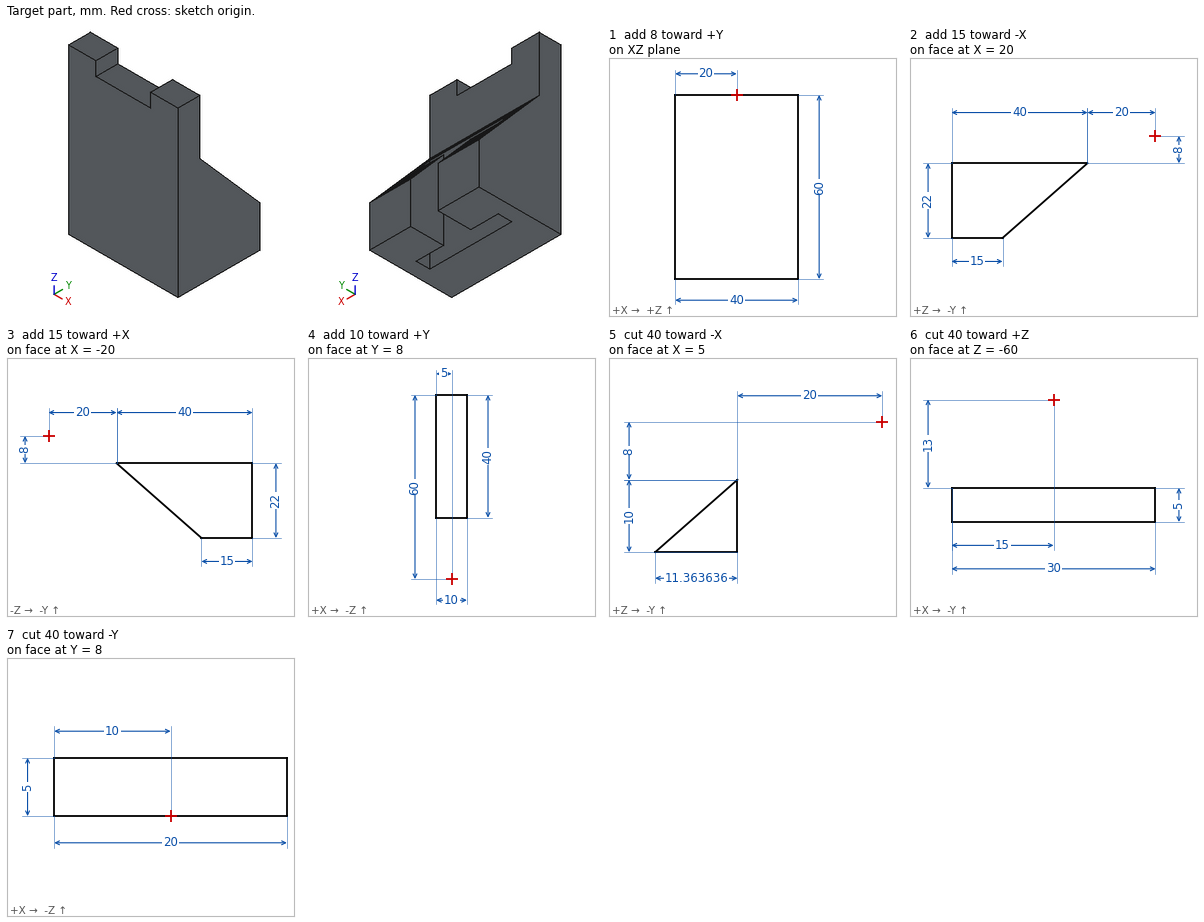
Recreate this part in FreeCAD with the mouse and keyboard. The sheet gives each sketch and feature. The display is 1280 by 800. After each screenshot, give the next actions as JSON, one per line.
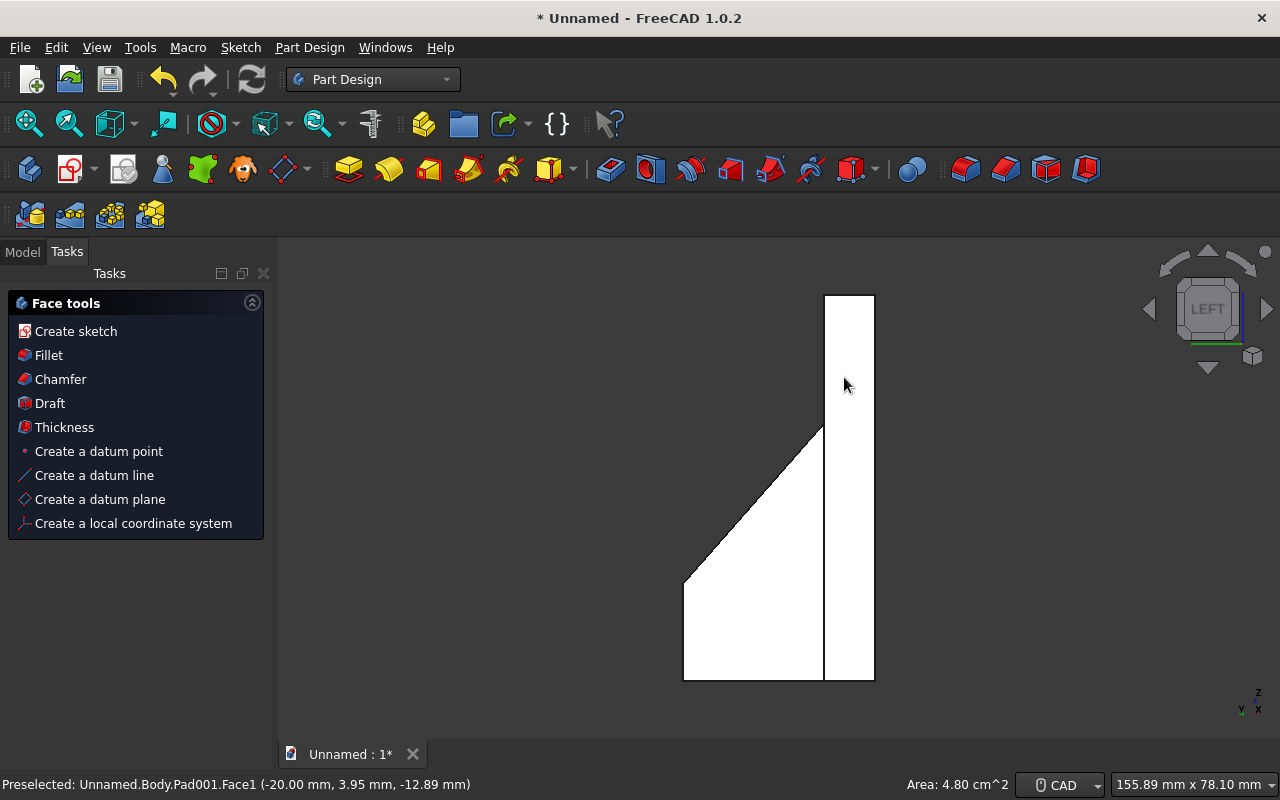
{"action": "left_click", "coordinate": [70, 170]}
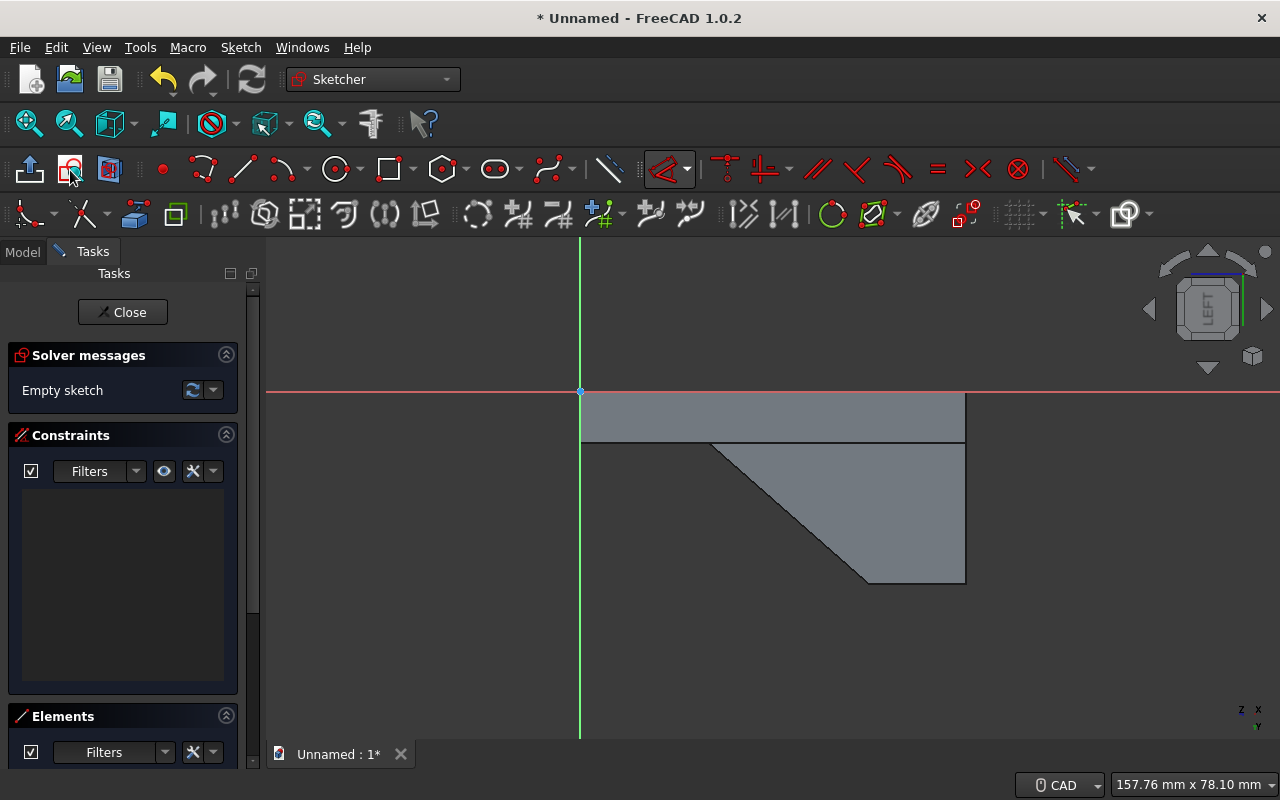
{"action": "scroll", "coordinate": [912, 488], "scroll_direction": "up", "scroll_amount": 2}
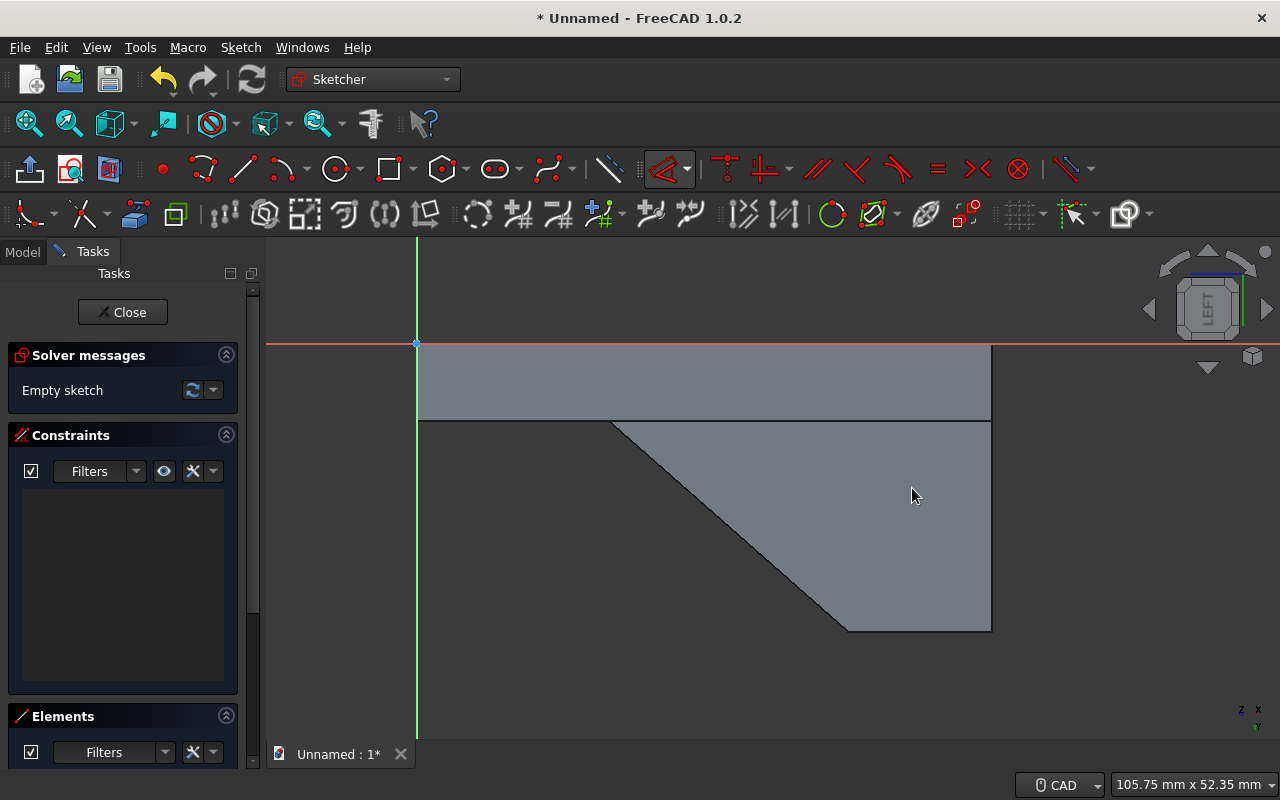
{"action": "left_click", "coordinate": [204, 170]}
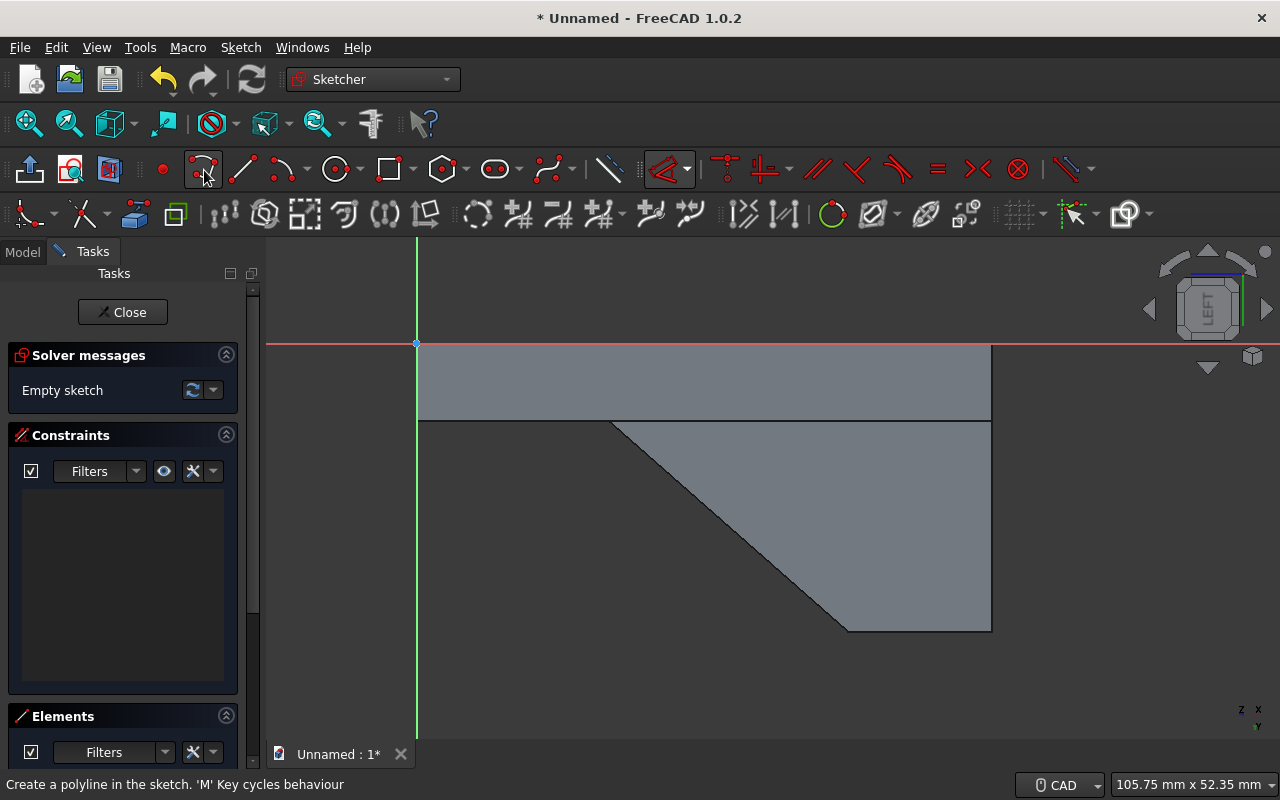
{"action": "left_click", "coordinate": [608, 421]}
{"action": "left_click", "coordinate": [848, 632]}
{"action": "left_click", "coordinate": [992, 632]}
{"action": "left_click", "coordinate": [992, 421]}
{"action": "left_click", "coordinate": [608, 422]}
{"action": "key", "text": "Escape"}
{"action": "key", "text": "Escape"}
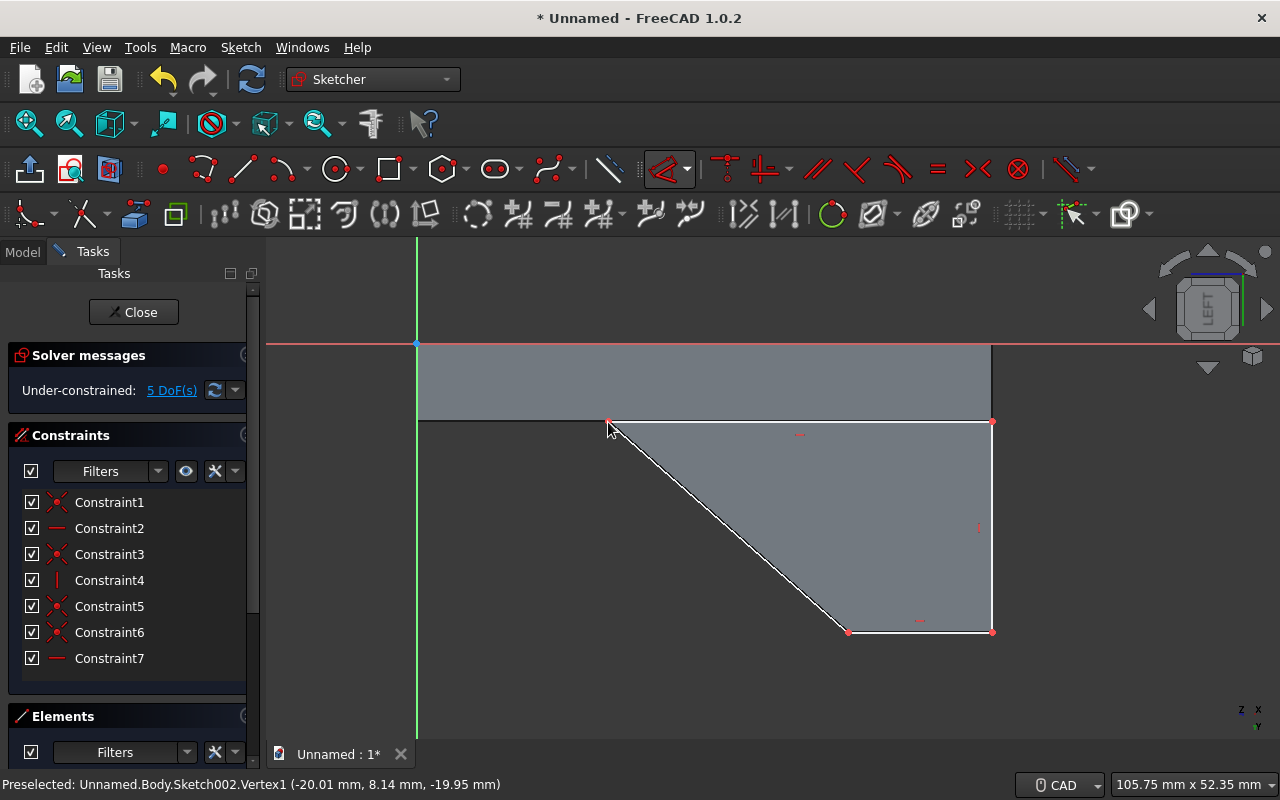
{"action": "left_click", "coordinate": [891, 633]}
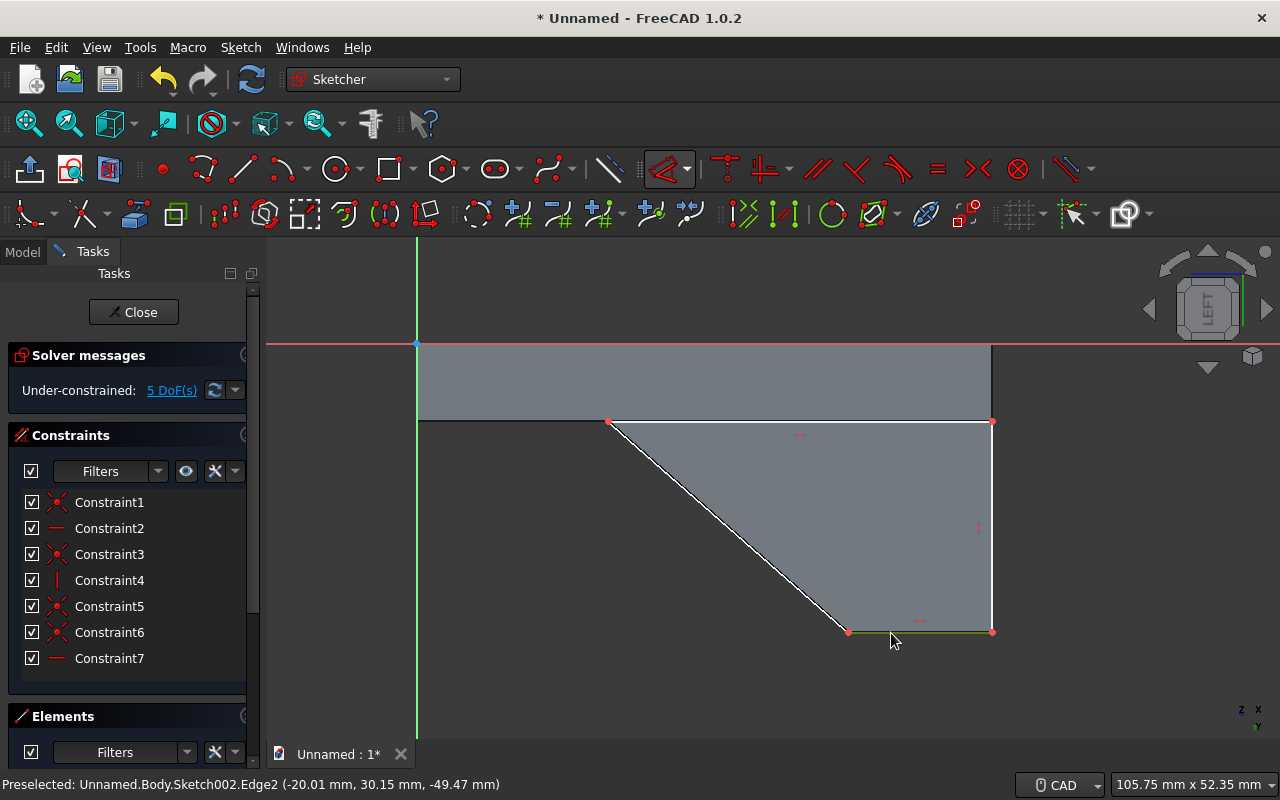
{"action": "left_click", "coordinate": [690, 170]}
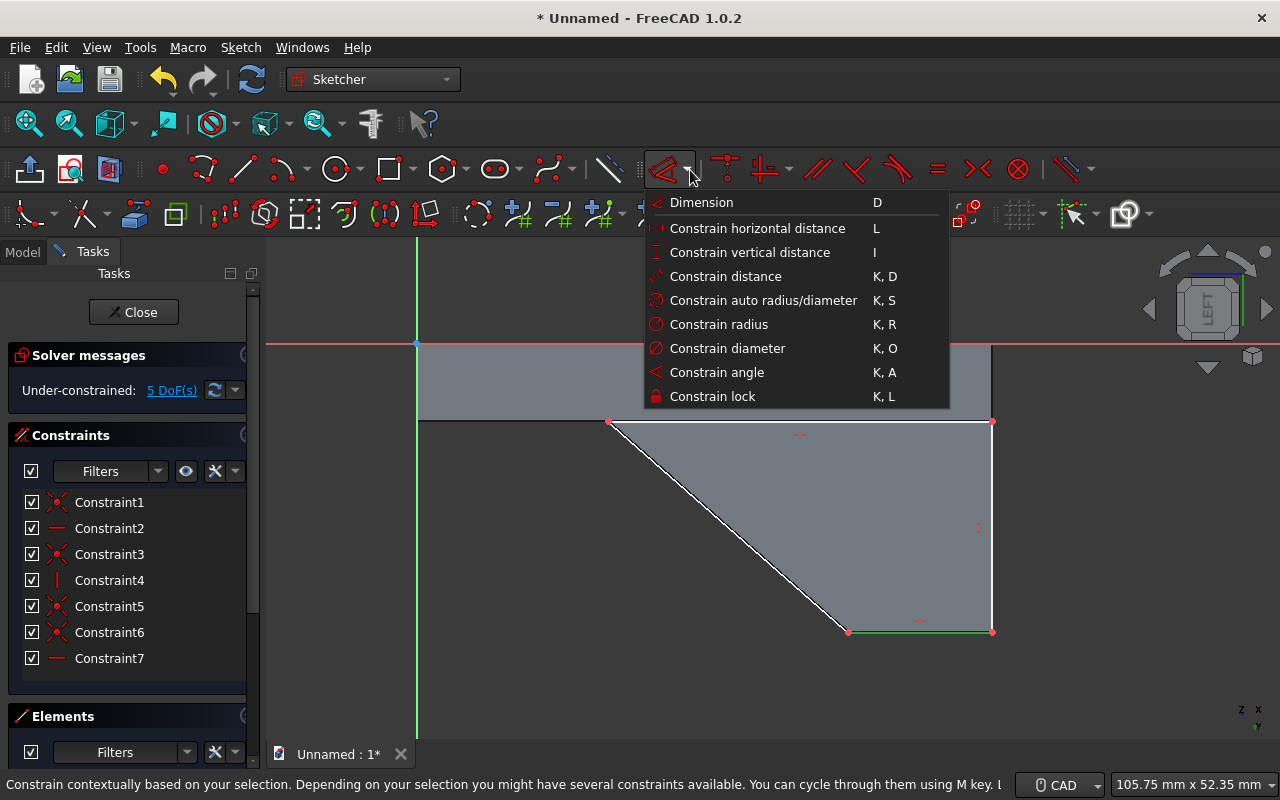
{"action": "left_click", "coordinate": [797, 228]}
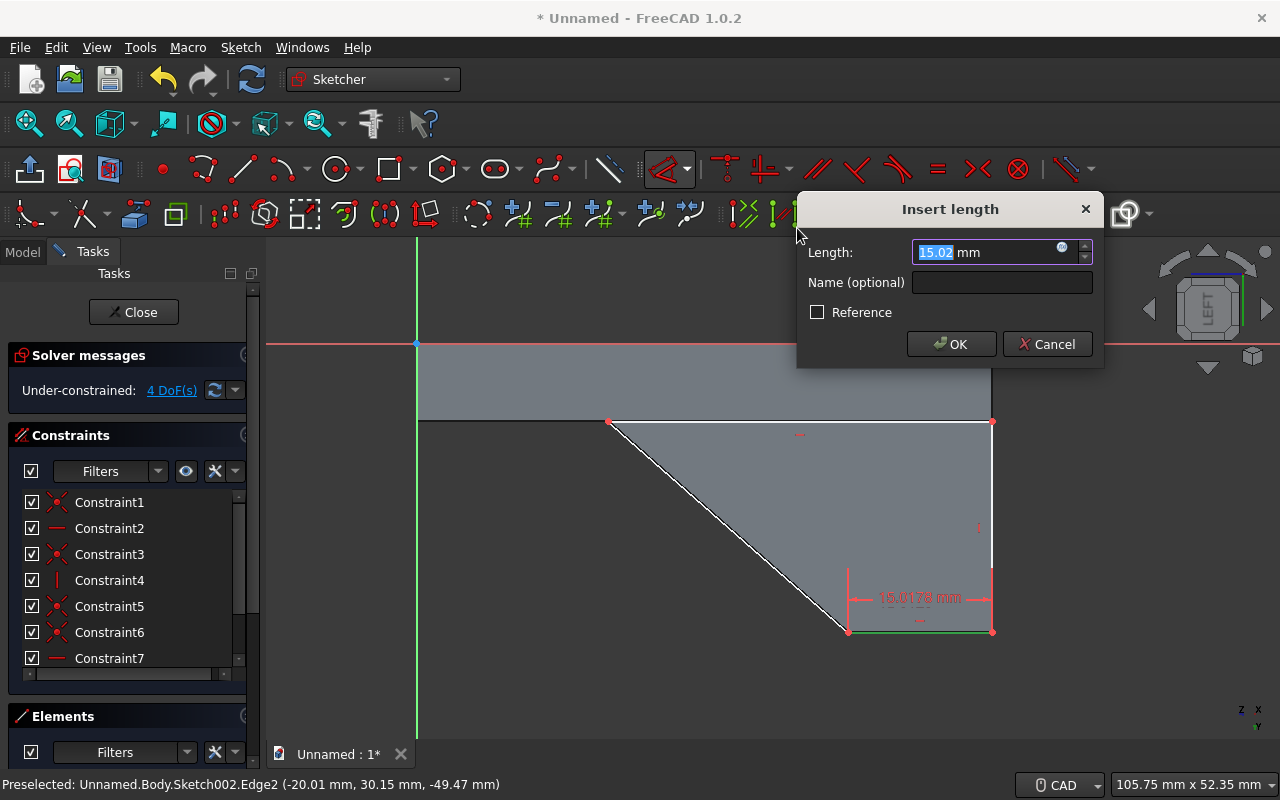
{"action": "type", "text": "15"}
{"action": "key", "text": "Return"}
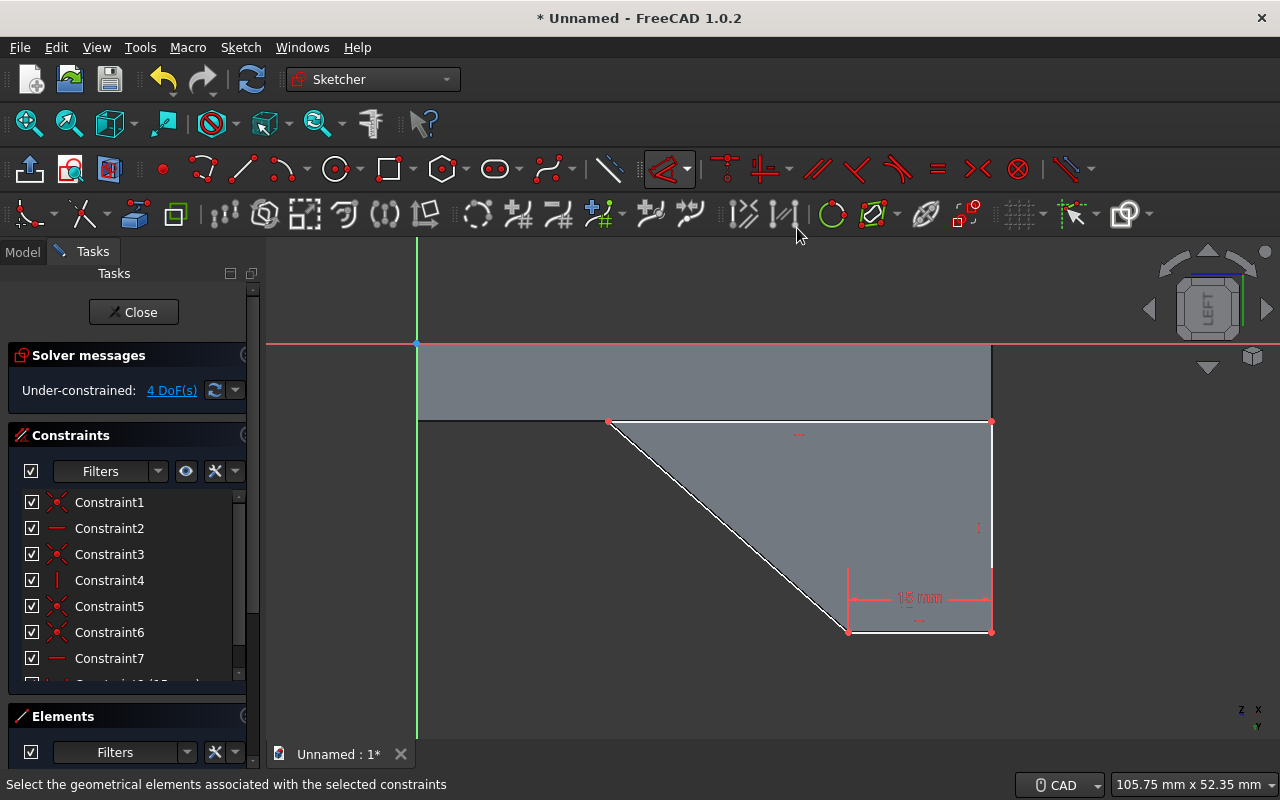
{"action": "left_click", "coordinate": [992, 570]}